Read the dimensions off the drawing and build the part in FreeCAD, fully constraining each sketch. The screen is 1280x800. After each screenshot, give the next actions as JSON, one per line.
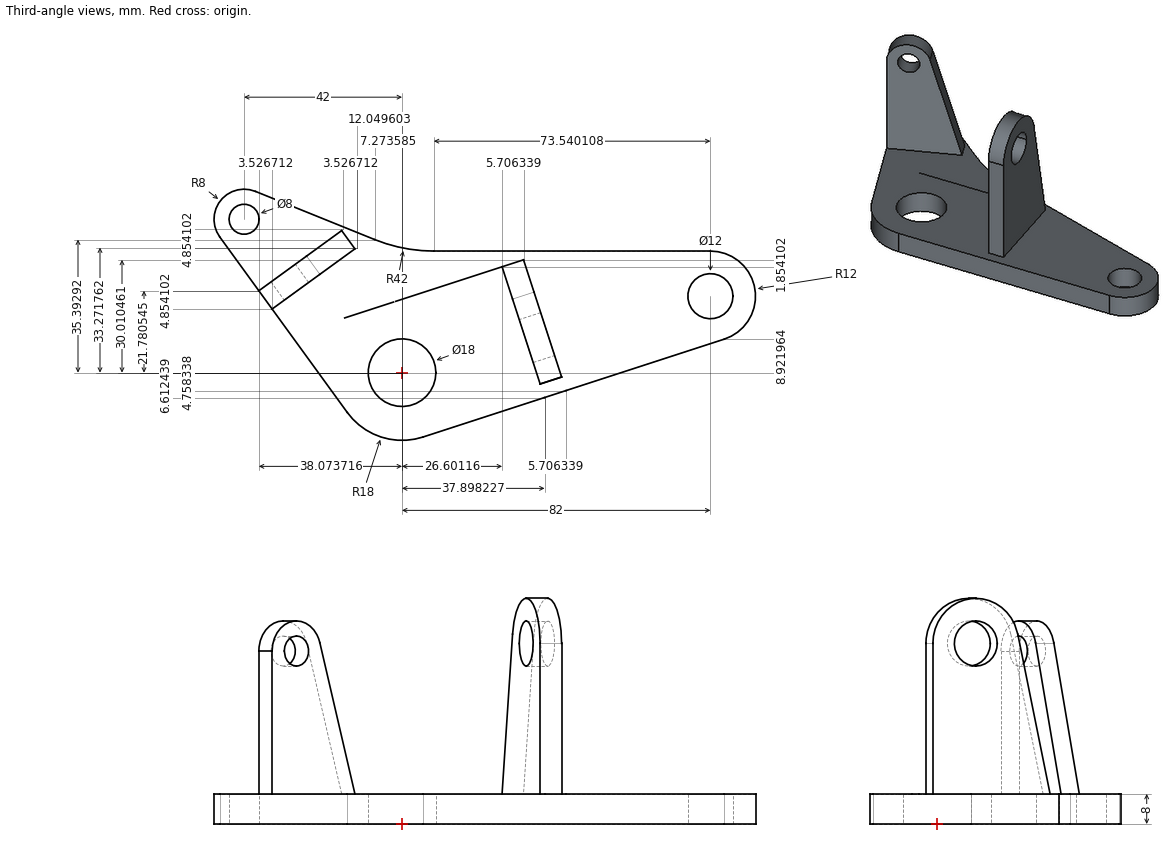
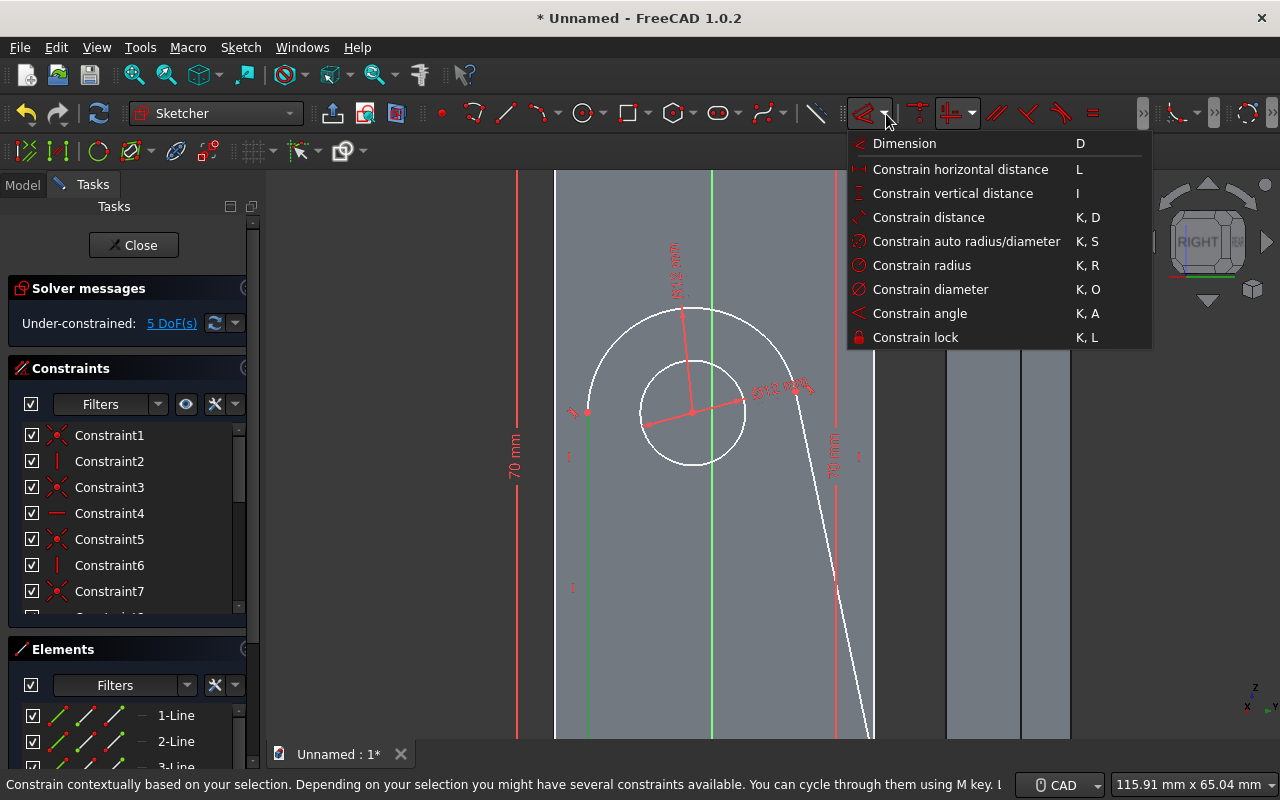
{"action": "left_click", "coordinate": [1000, 193]}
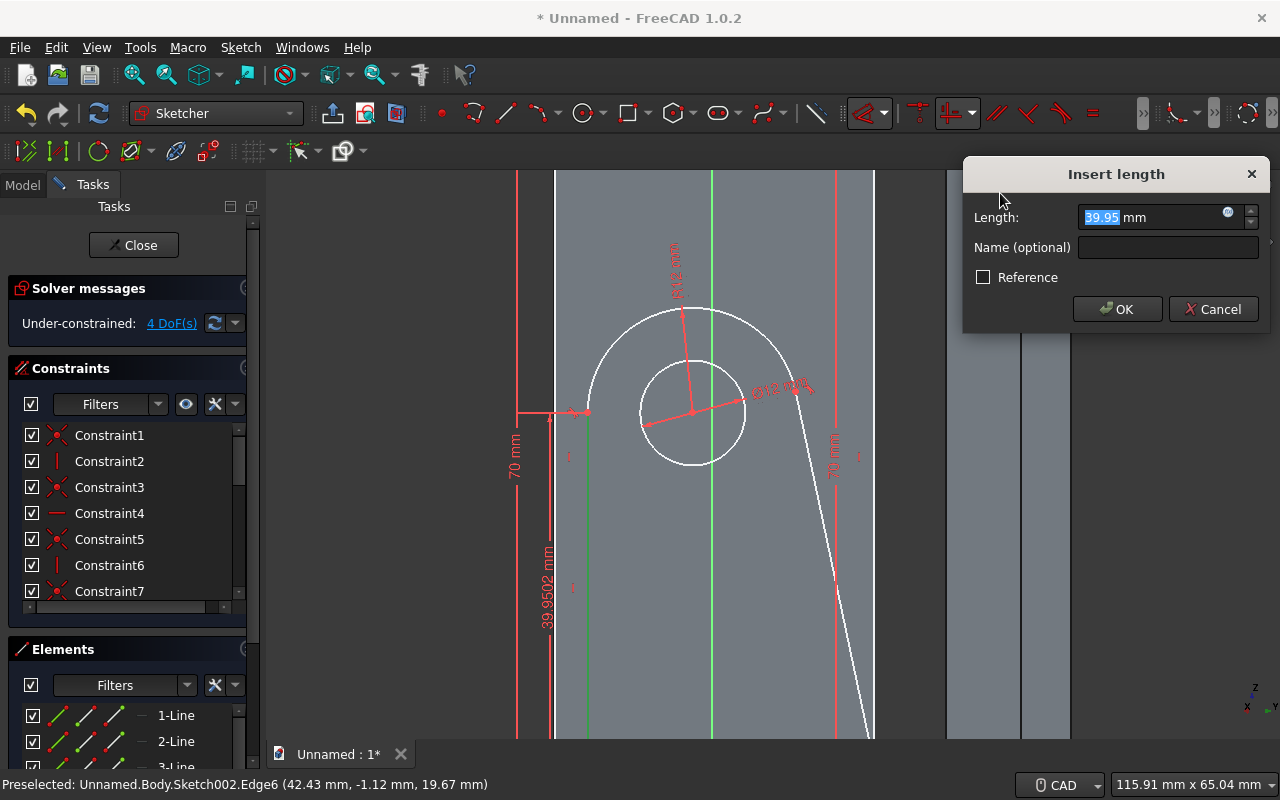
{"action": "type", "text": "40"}
{"action": "key", "text": "Return"}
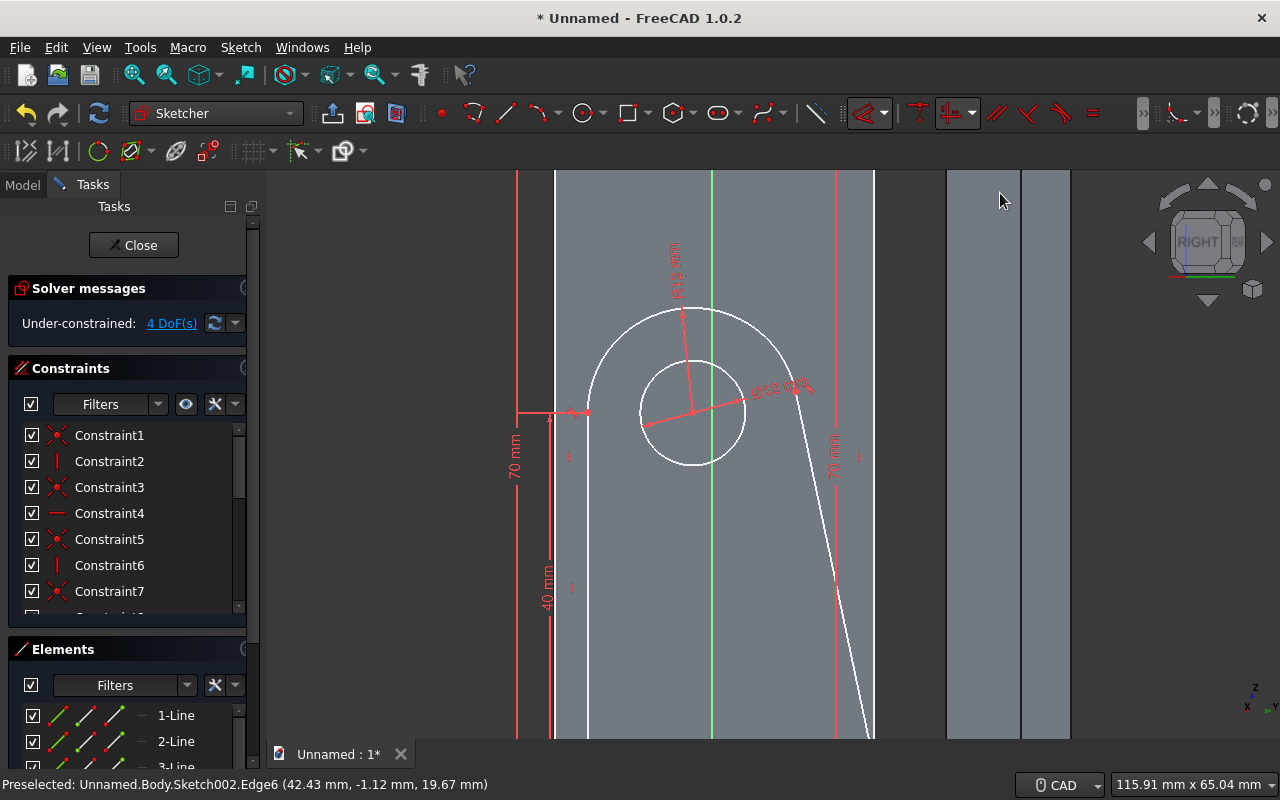
{"action": "scroll", "coordinate": [693, 411], "scroll_direction": "down", "scroll_amount": 3}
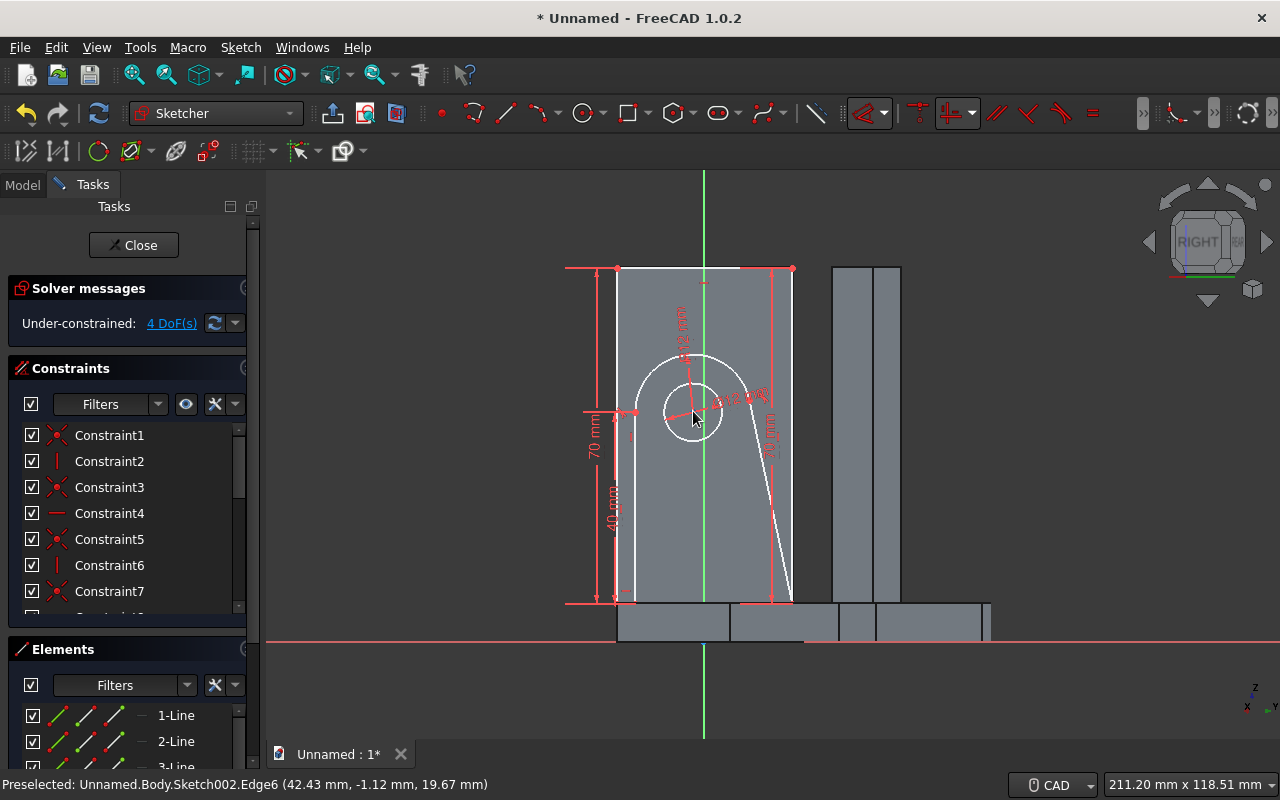
{"action": "left_click", "coordinate": [792, 604]}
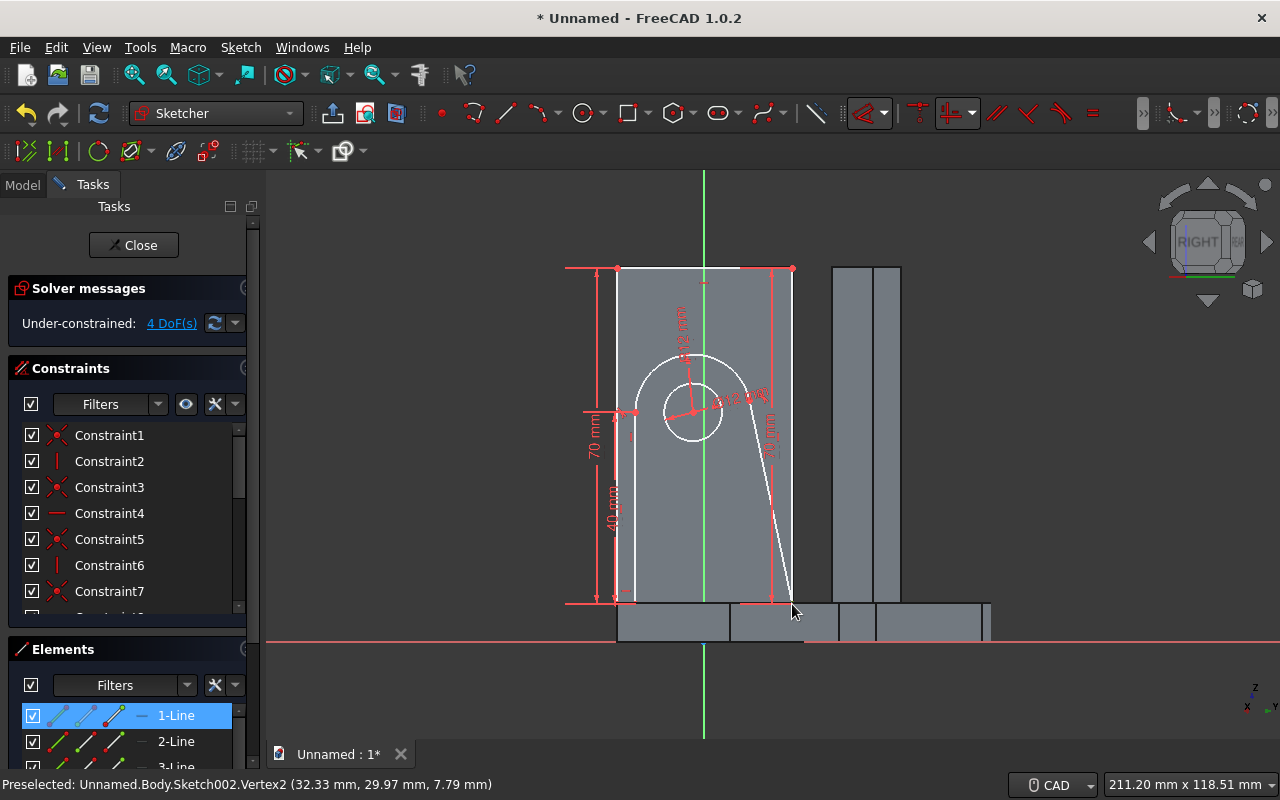
{"action": "key", "text": "i"}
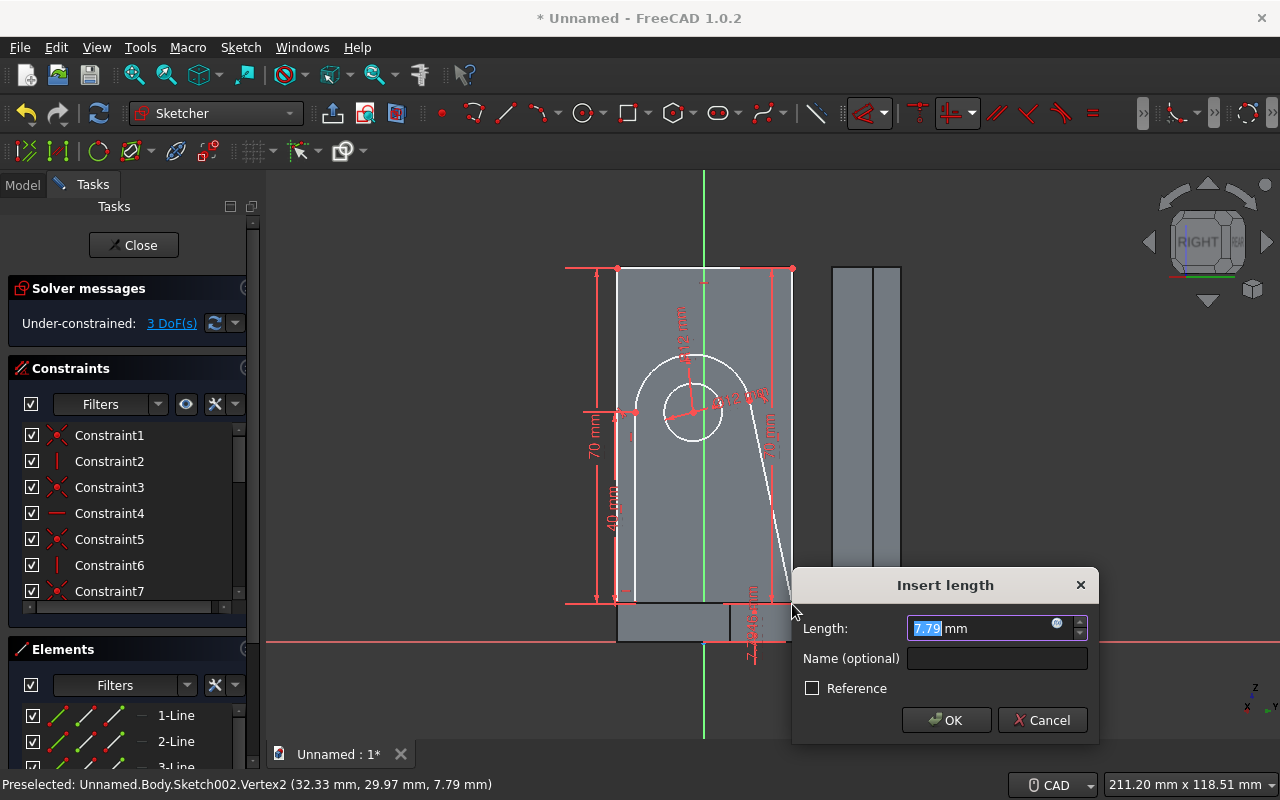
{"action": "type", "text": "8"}
{"action": "key", "text": "Return"}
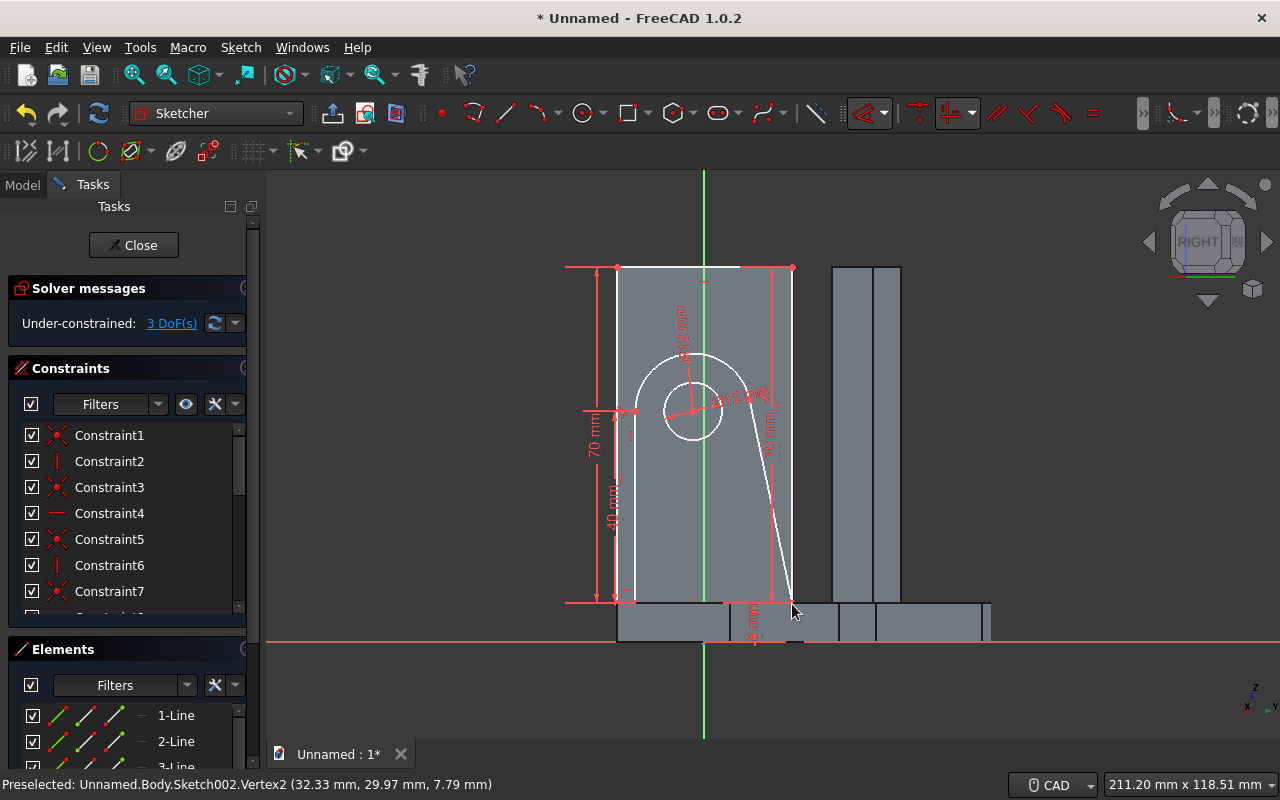
{"action": "scroll", "coordinate": [693, 411], "scroll_direction": "up", "scroll_amount": 7}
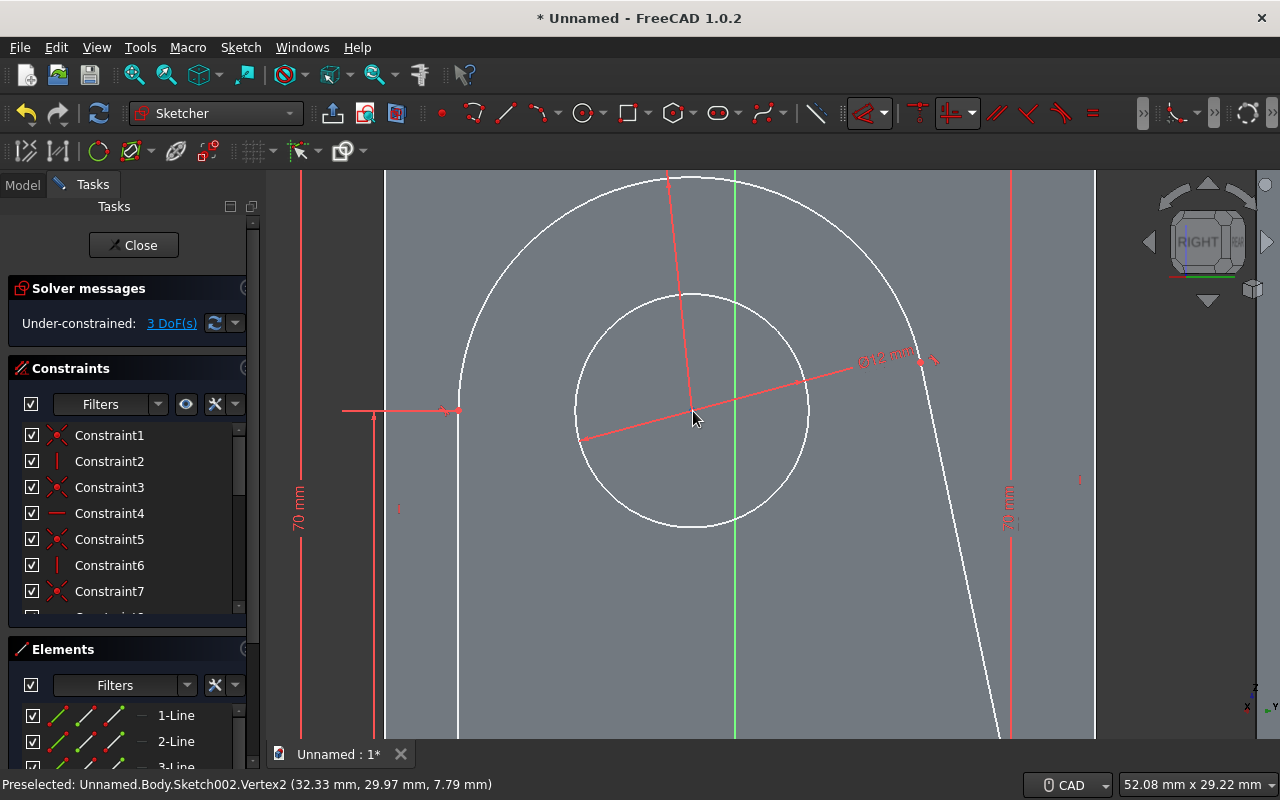
{"action": "left_click", "coordinate": [692, 411]}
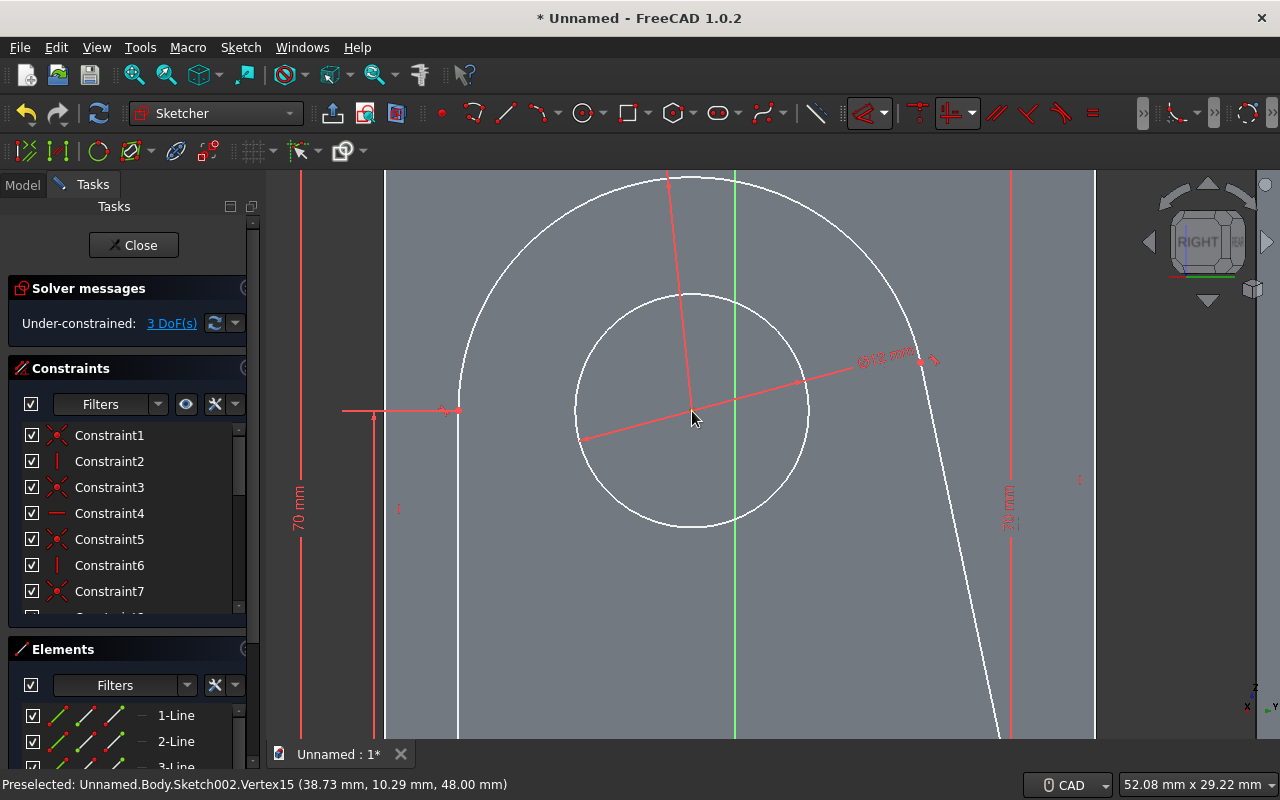
{"action": "key", "text": "l"}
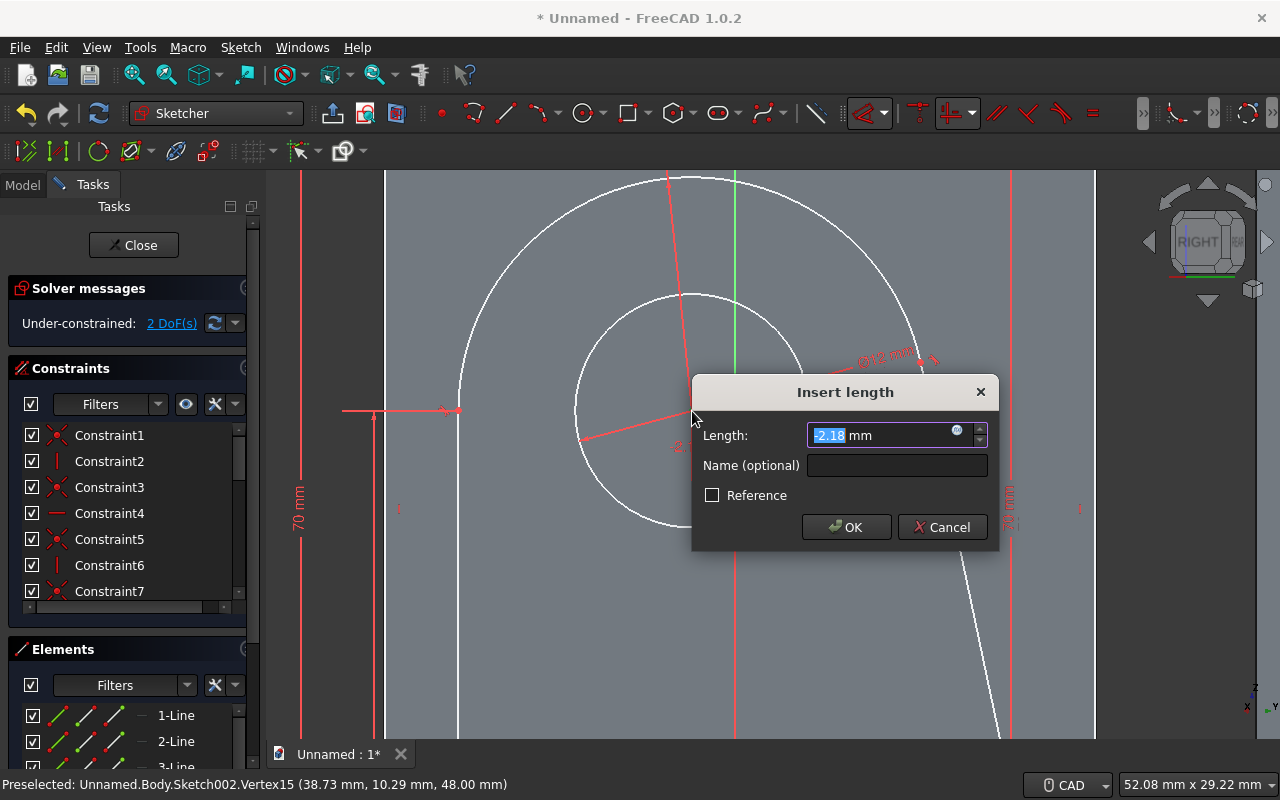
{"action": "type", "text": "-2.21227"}
{"action": "key", "text": "Return"}